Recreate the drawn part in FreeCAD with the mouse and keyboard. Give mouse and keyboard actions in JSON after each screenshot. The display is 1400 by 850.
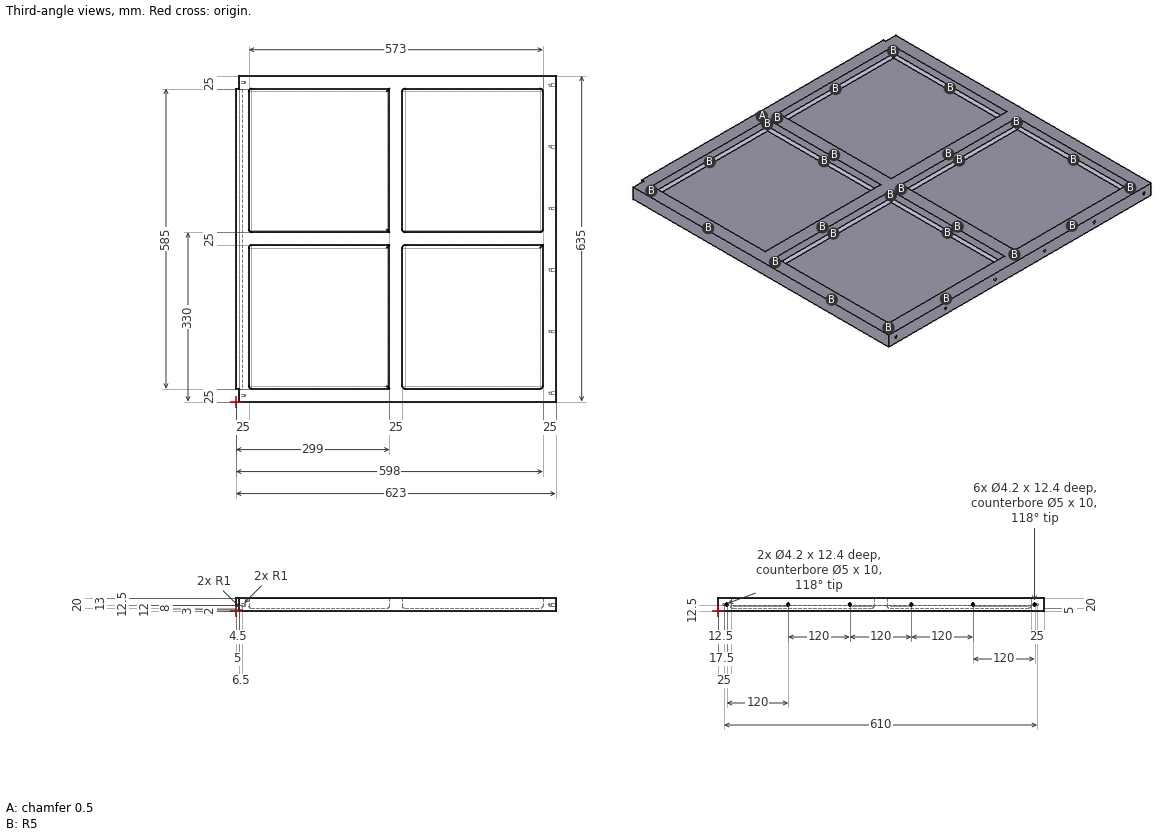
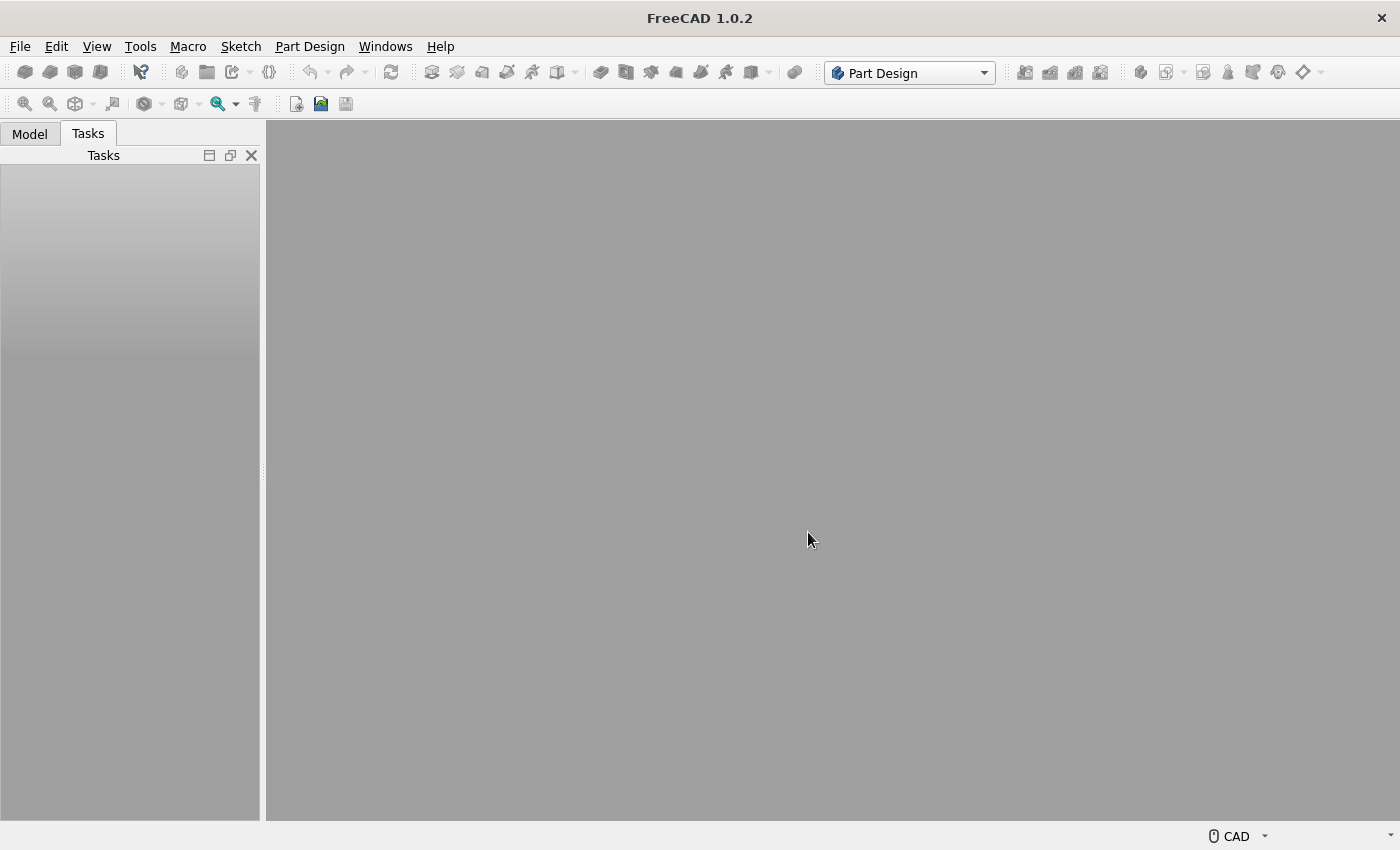
{"action": "left_click", "coordinate": [296, 104]}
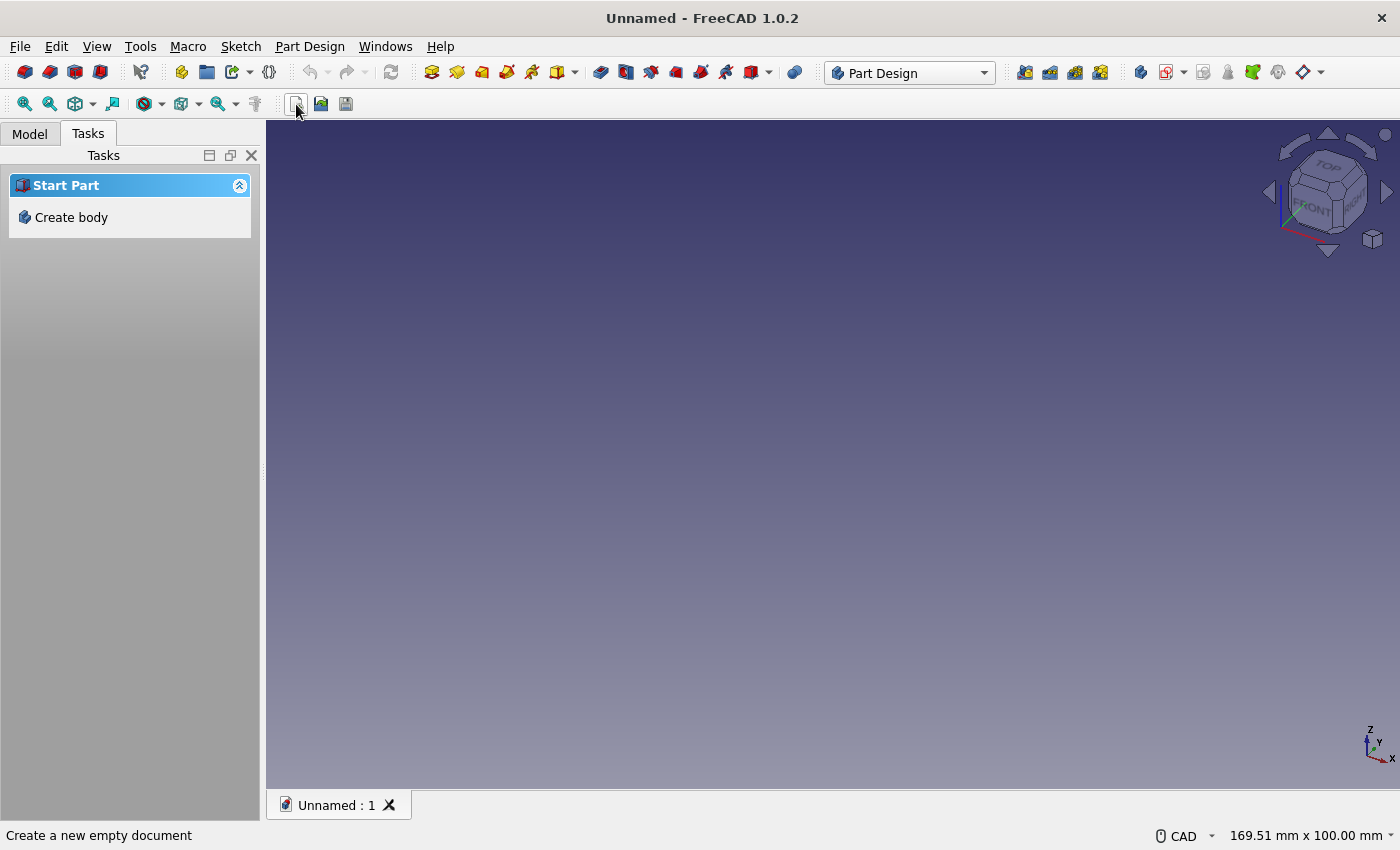
{"action": "left_click", "coordinate": [1166, 72]}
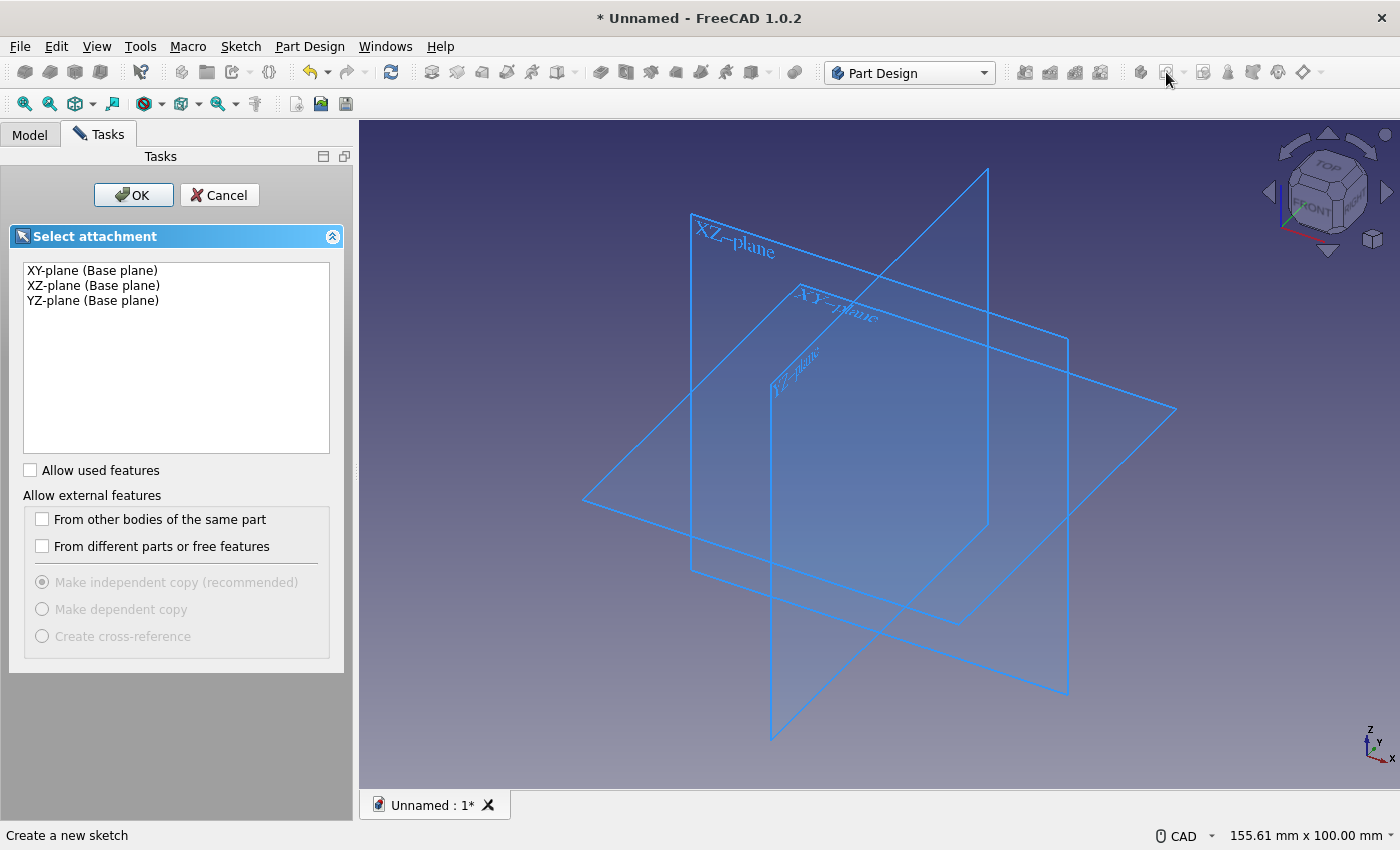
{"action": "left_click", "coordinate": [84, 270]}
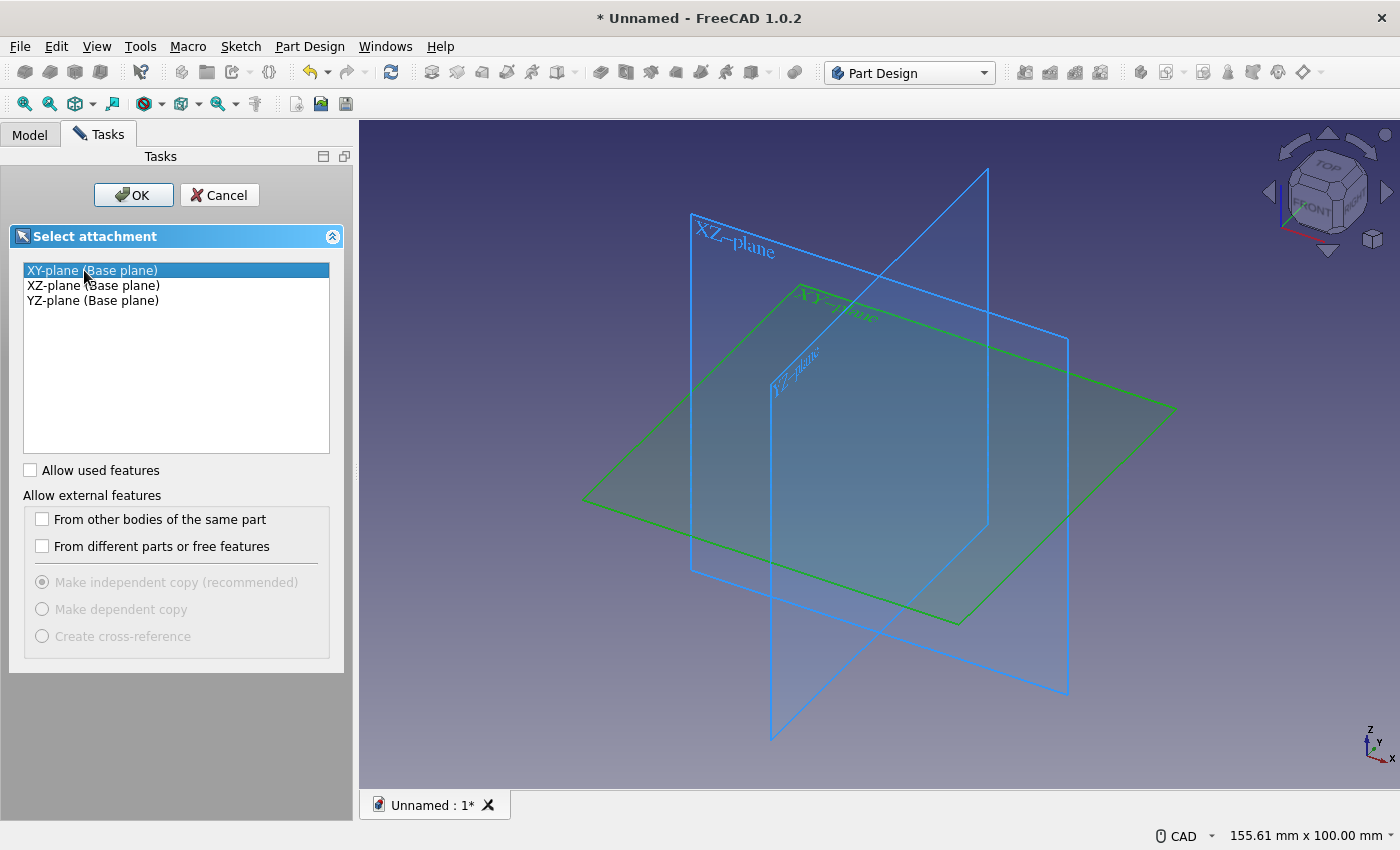
{"action": "left_click", "coordinate": [134, 195]}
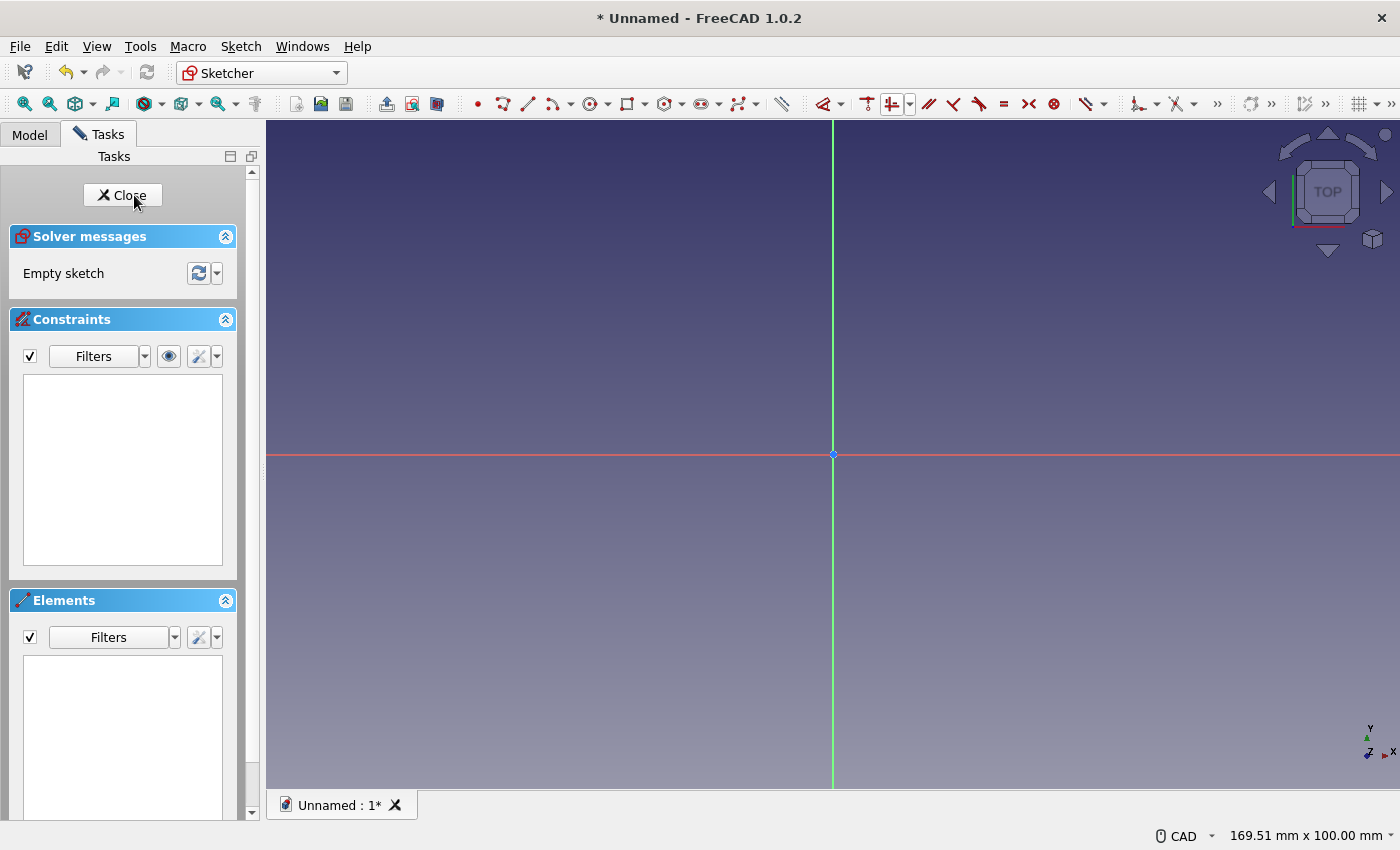
{"action": "scroll", "coordinate": [496, 719], "scroll_direction": "down", "scroll_amount": 11}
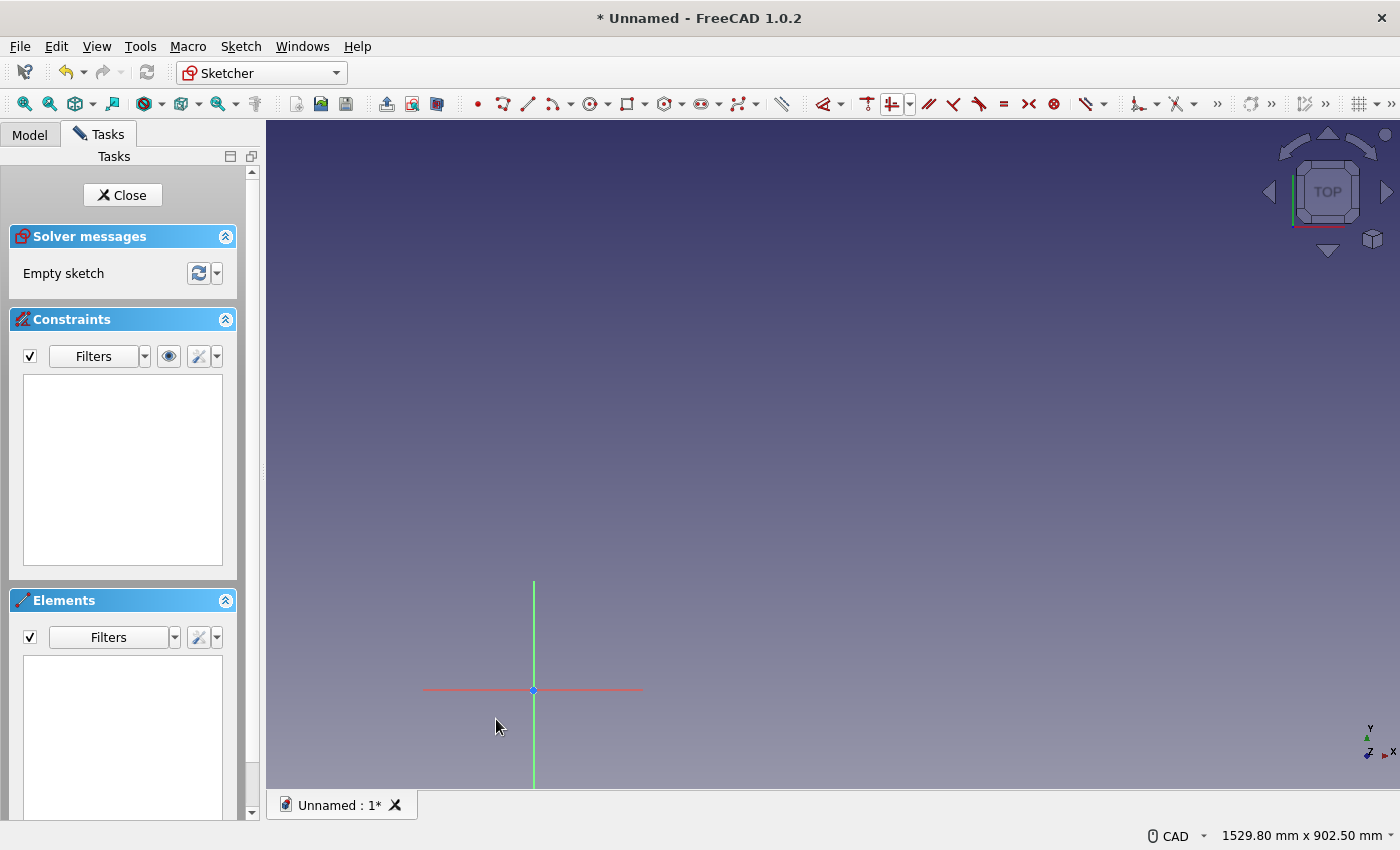
{"action": "left_click", "coordinate": [626, 104]}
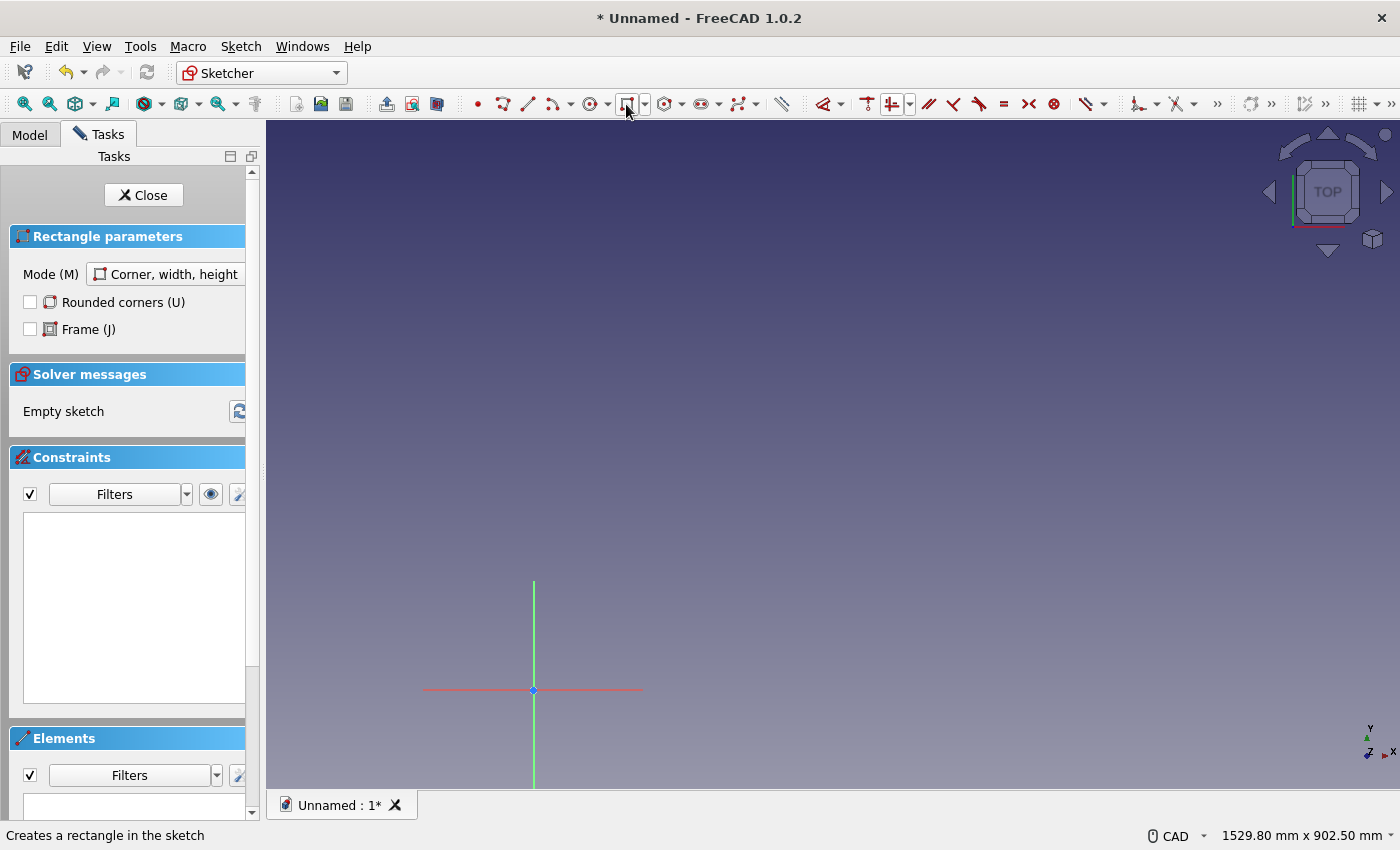
{"action": "left_click", "coordinate": [534, 690]}
{"action": "left_click", "coordinate": [995, 220]}
{"action": "key", "text": "Escape"}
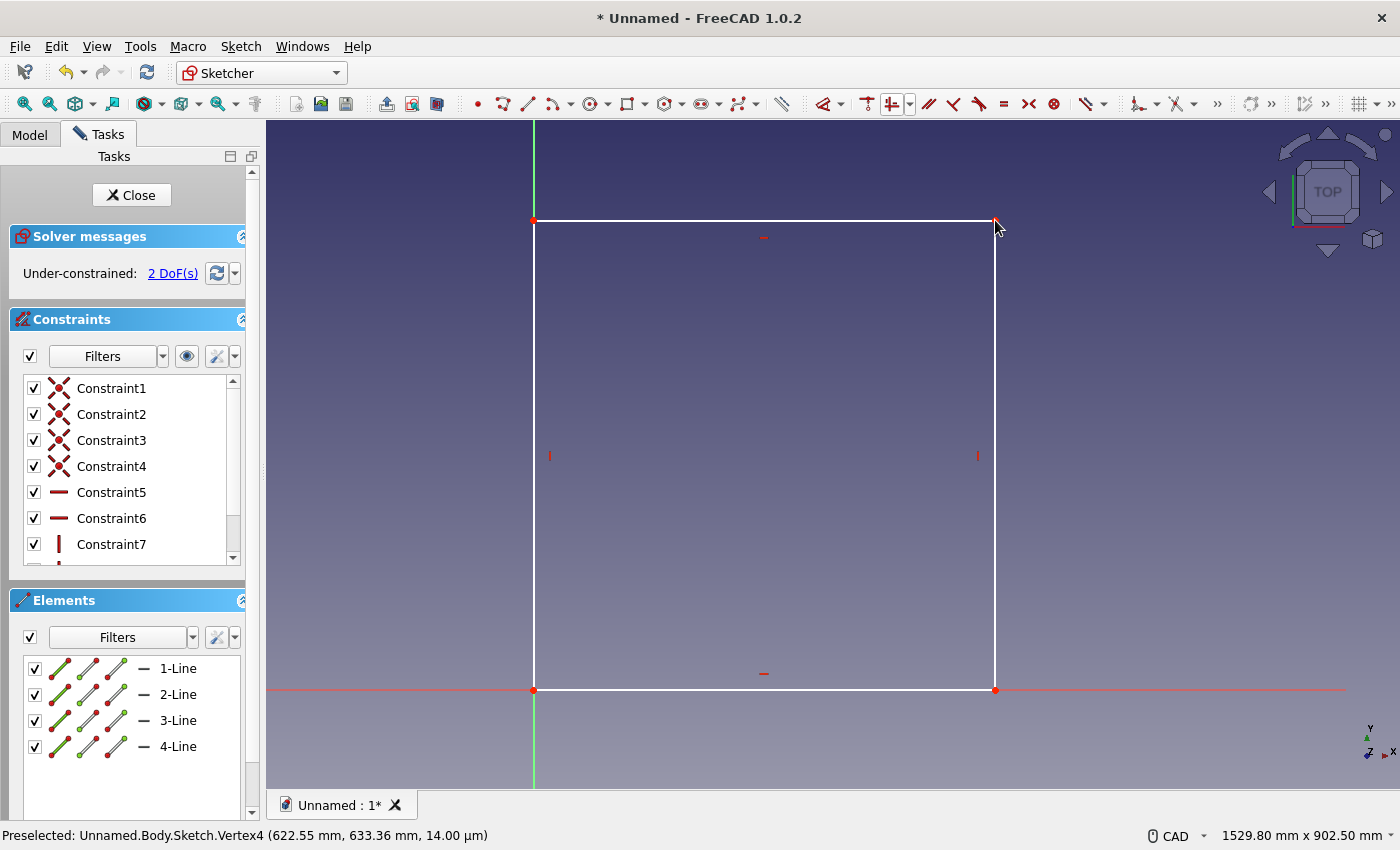
{"action": "left_click", "coordinate": [822, 104]}